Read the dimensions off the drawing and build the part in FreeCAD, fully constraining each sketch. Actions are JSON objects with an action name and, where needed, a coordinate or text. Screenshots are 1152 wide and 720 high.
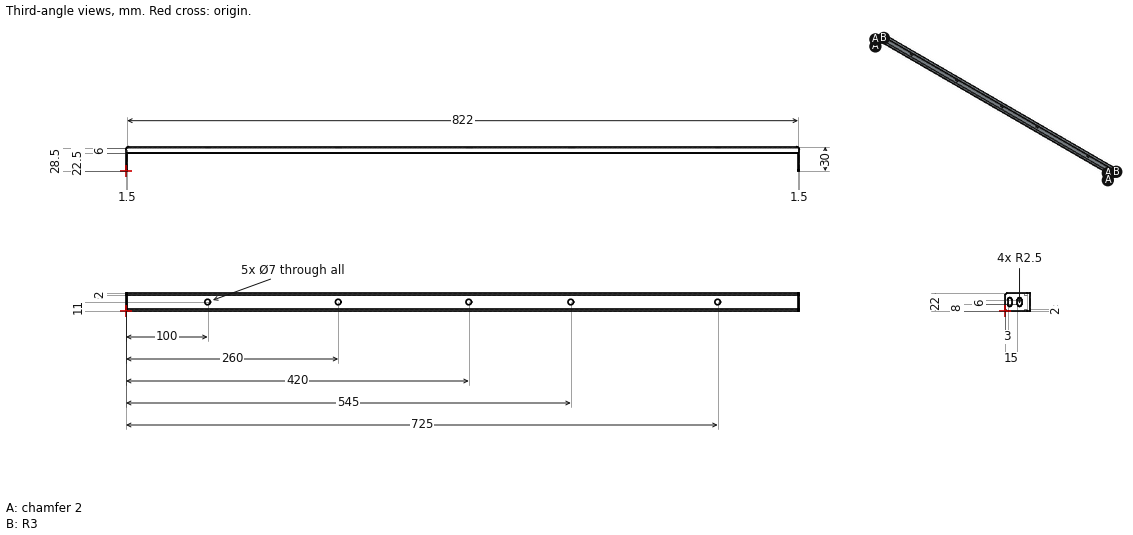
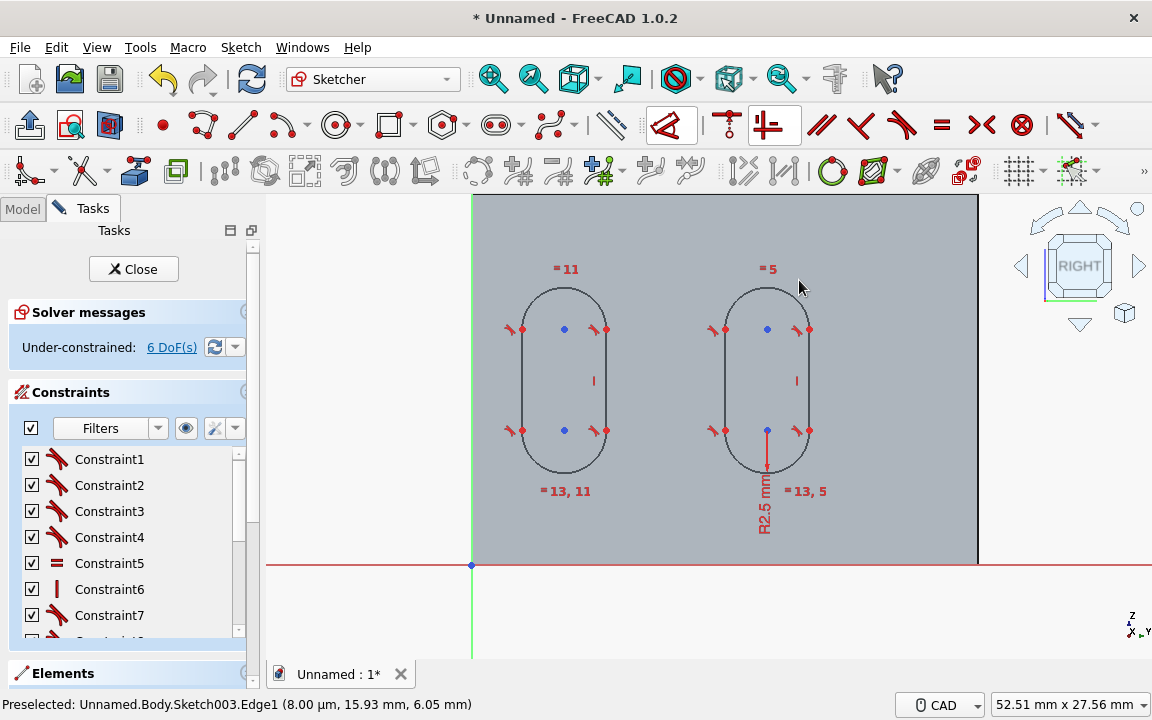
{"action": "left_click", "coordinate": [725, 401]}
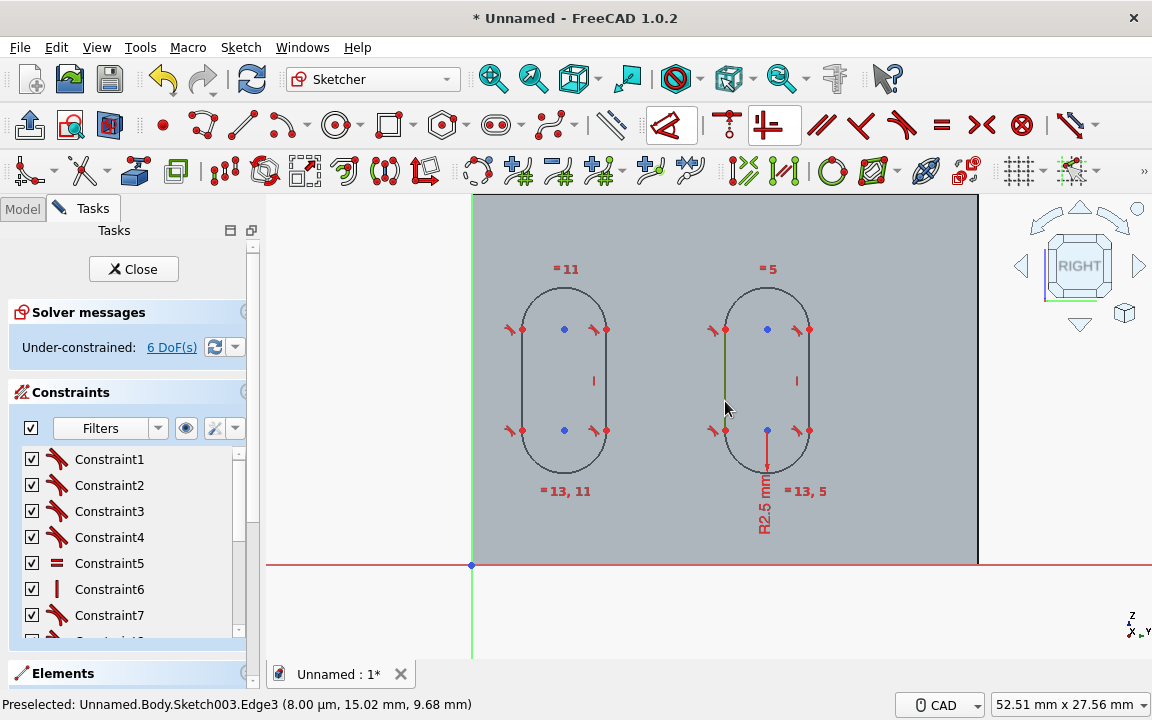
{"action": "key", "text": "i"}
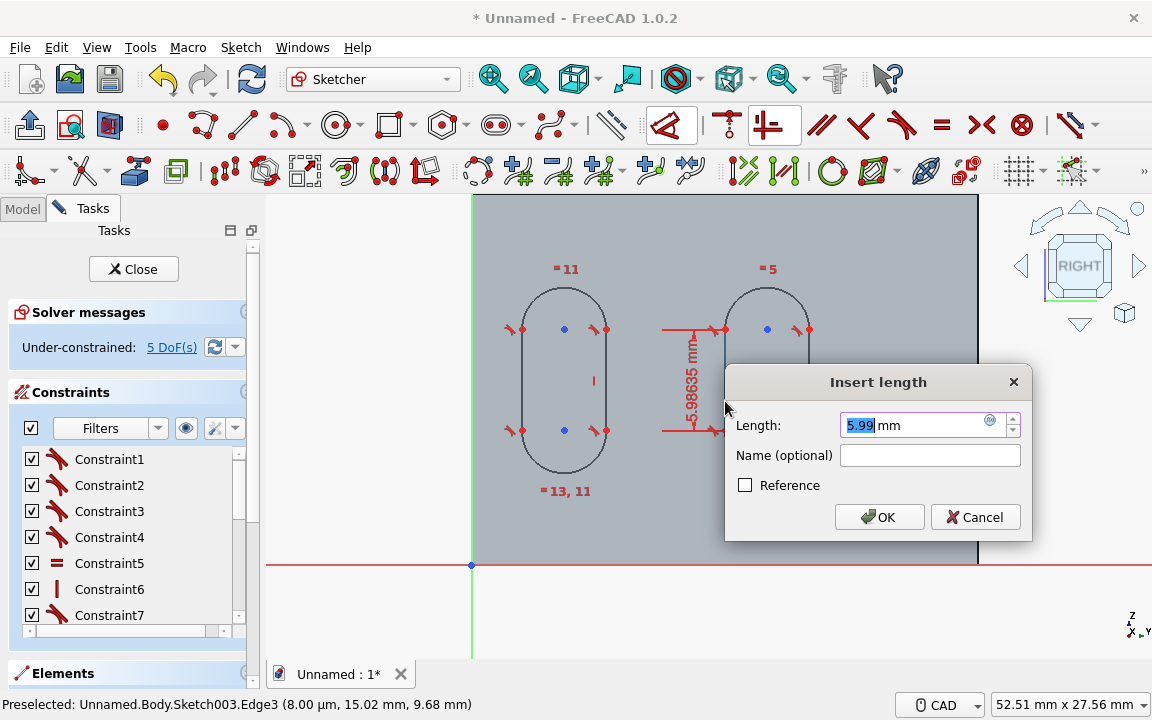
{"action": "type", "text": "6"}
{"action": "key", "text": "Return"}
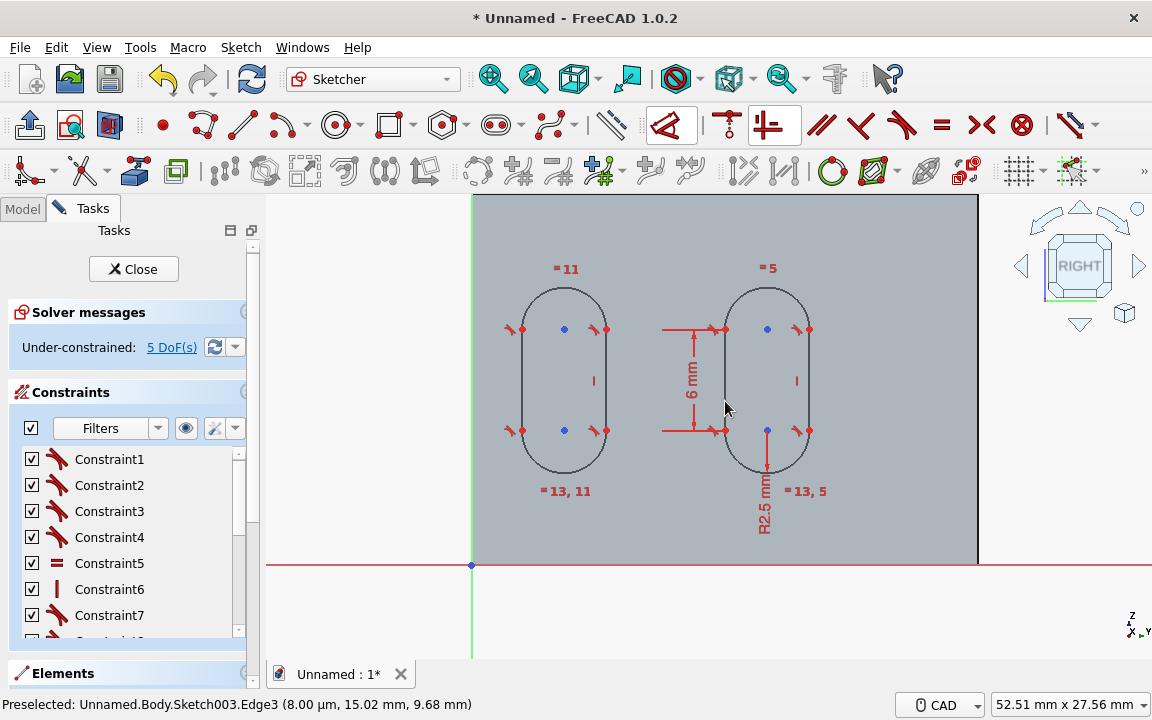
{"action": "left_click", "coordinate": [522, 401]}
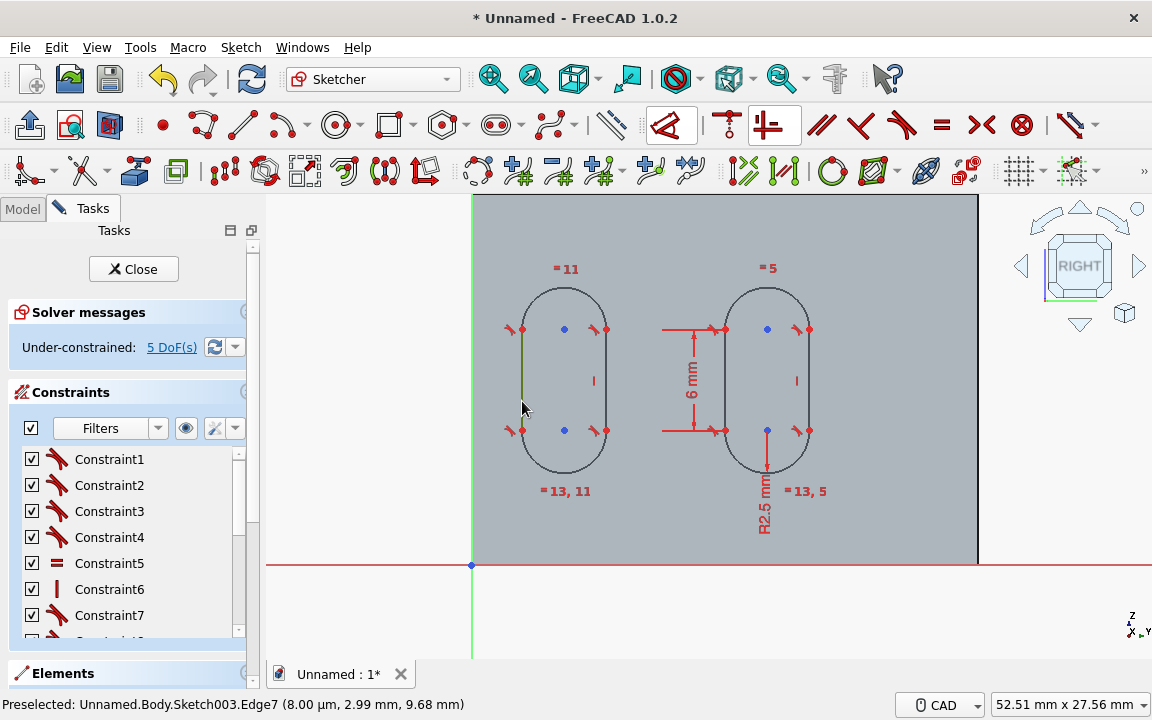
{"action": "key", "text": "i"}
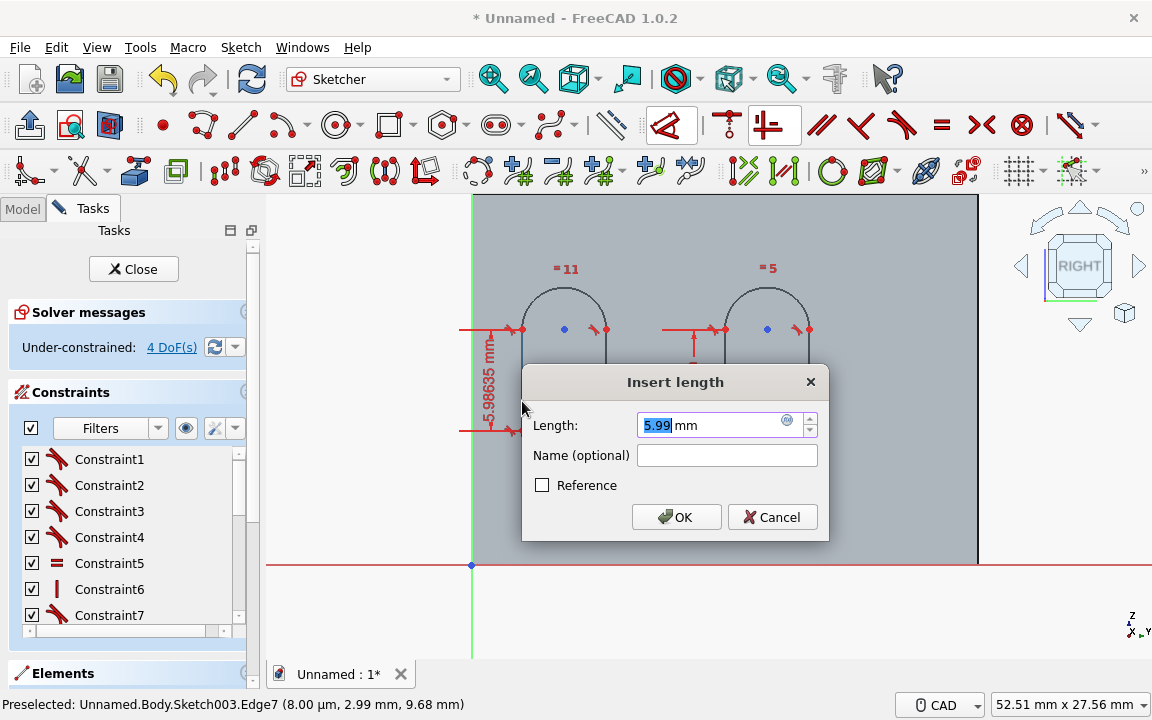
{"action": "type", "text": "6"}
{"action": "key", "text": "Return"}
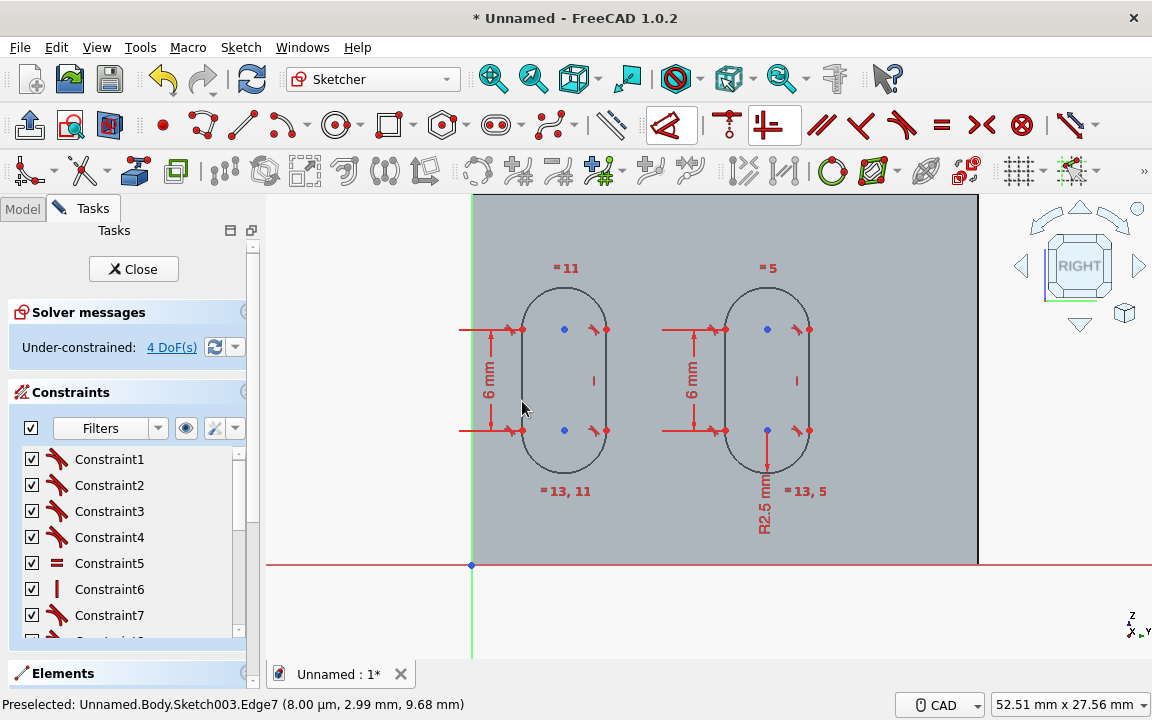
{"action": "left_click", "coordinate": [725, 431]}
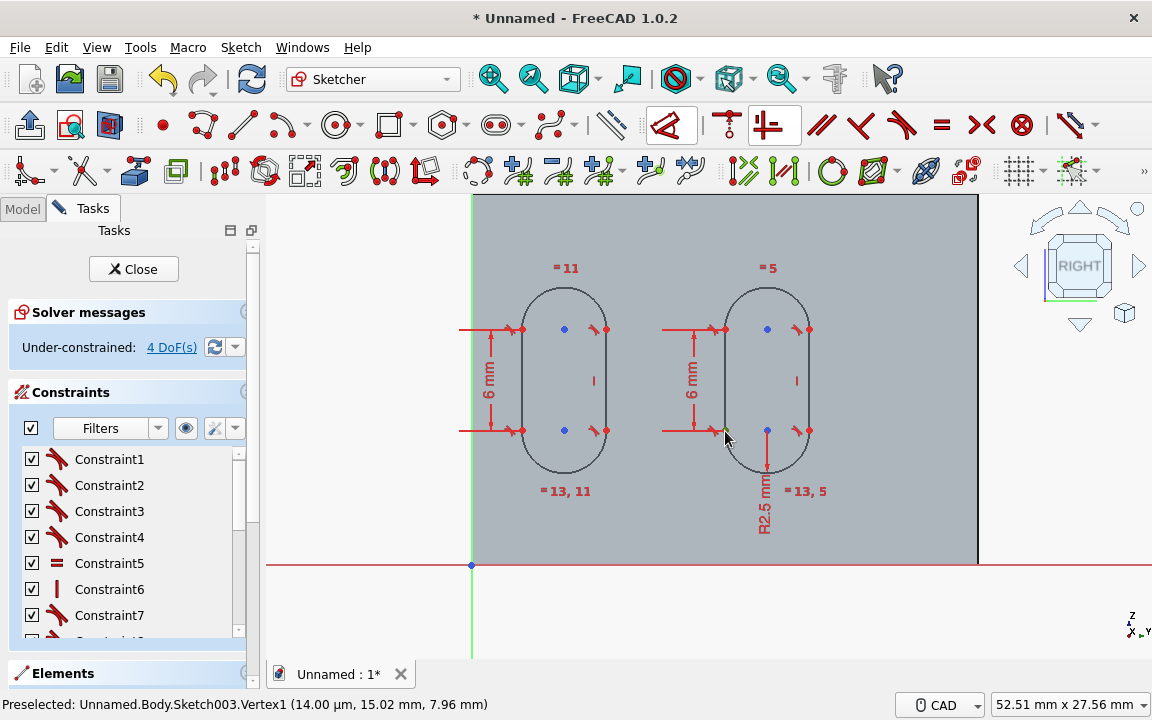
{"action": "left_click", "coordinate": [692, 126]}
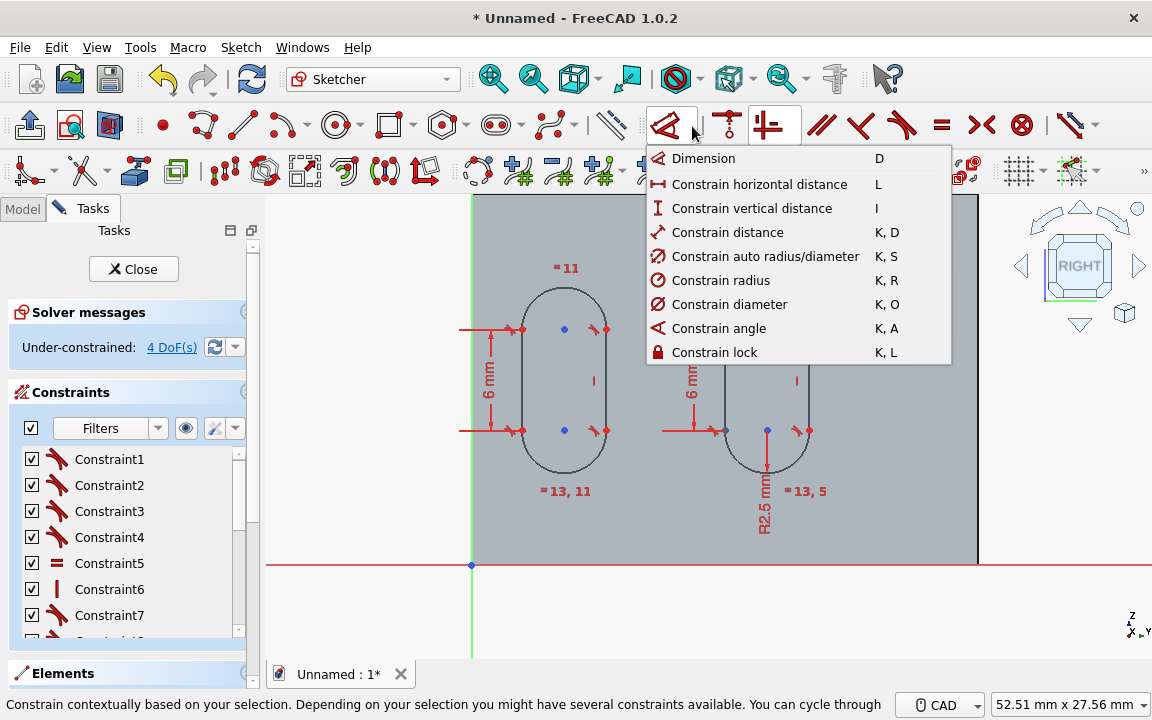
{"action": "left_click", "coordinate": [799, 208]}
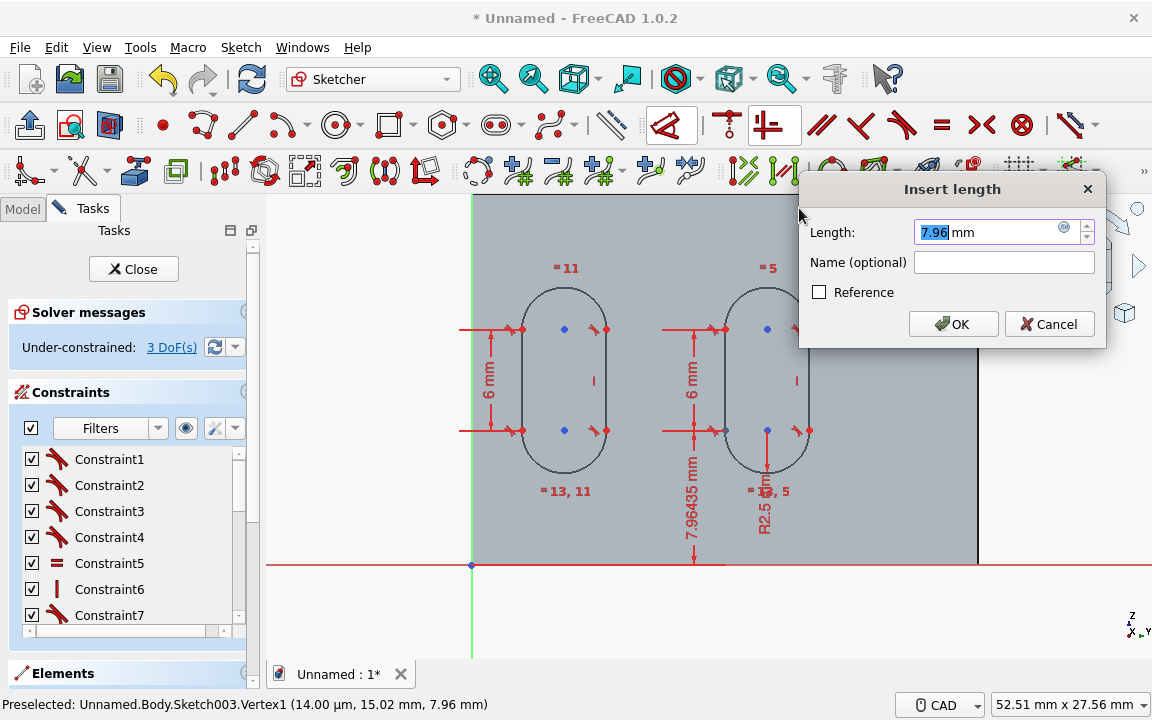
{"action": "type", "text": "8"}
{"action": "key", "text": "Return"}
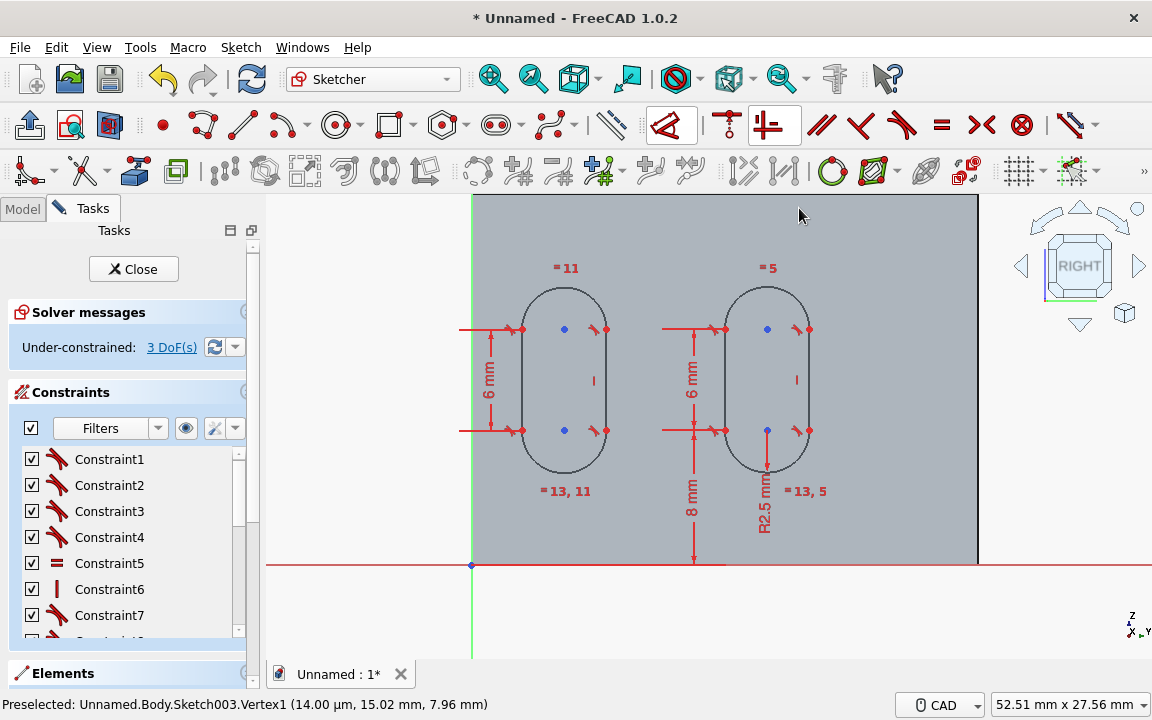
{"action": "left_click", "coordinate": [522, 431]}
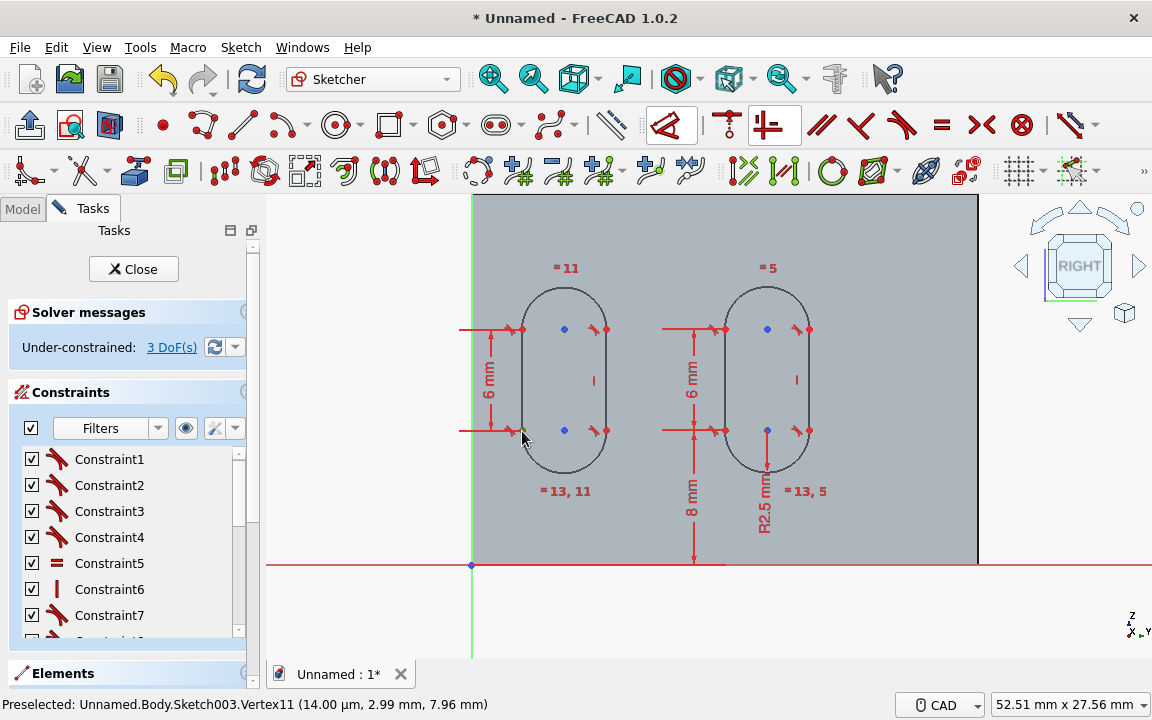
{"action": "key", "text": "l"}